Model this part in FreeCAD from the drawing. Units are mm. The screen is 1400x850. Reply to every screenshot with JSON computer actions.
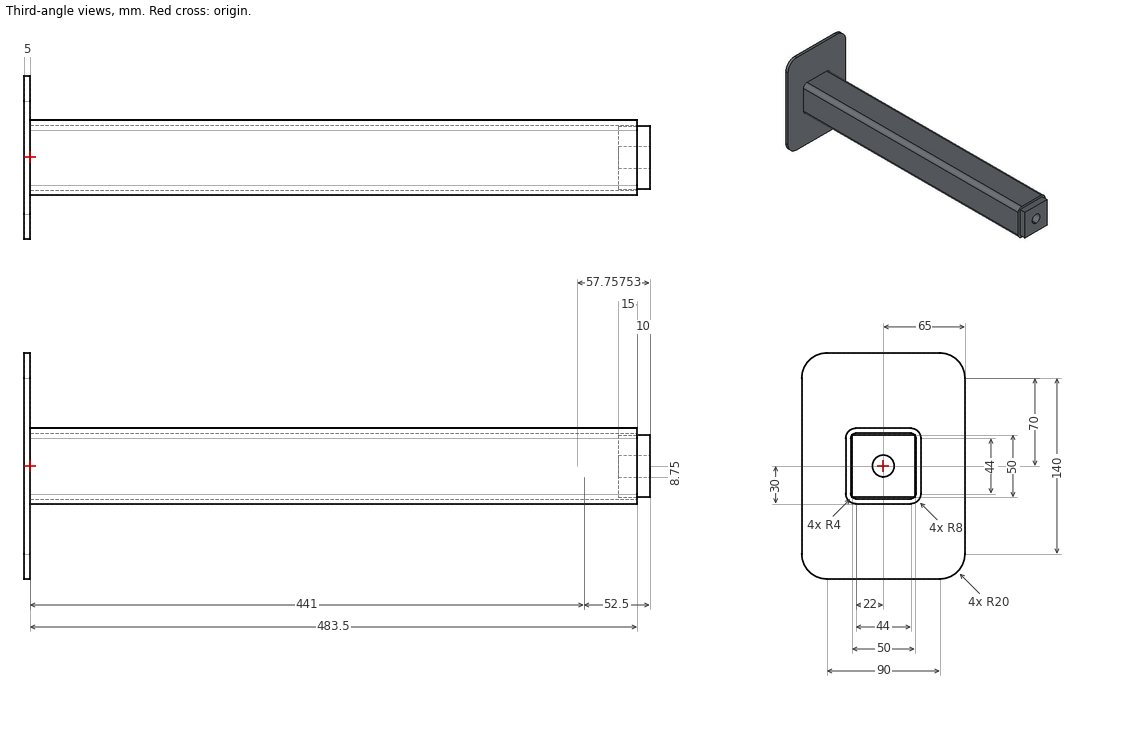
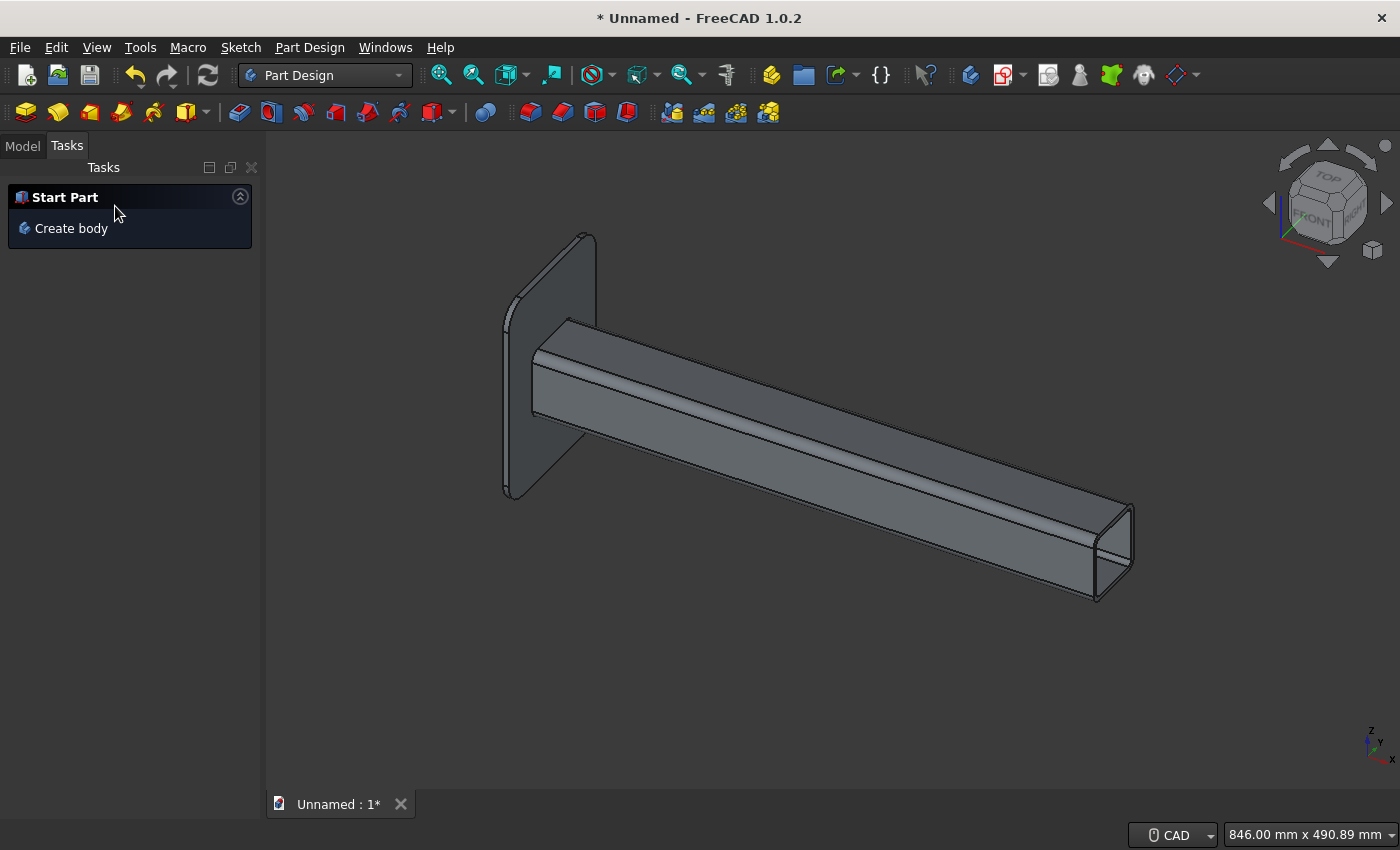
{"action": "left_click", "coordinate": [442, 76]}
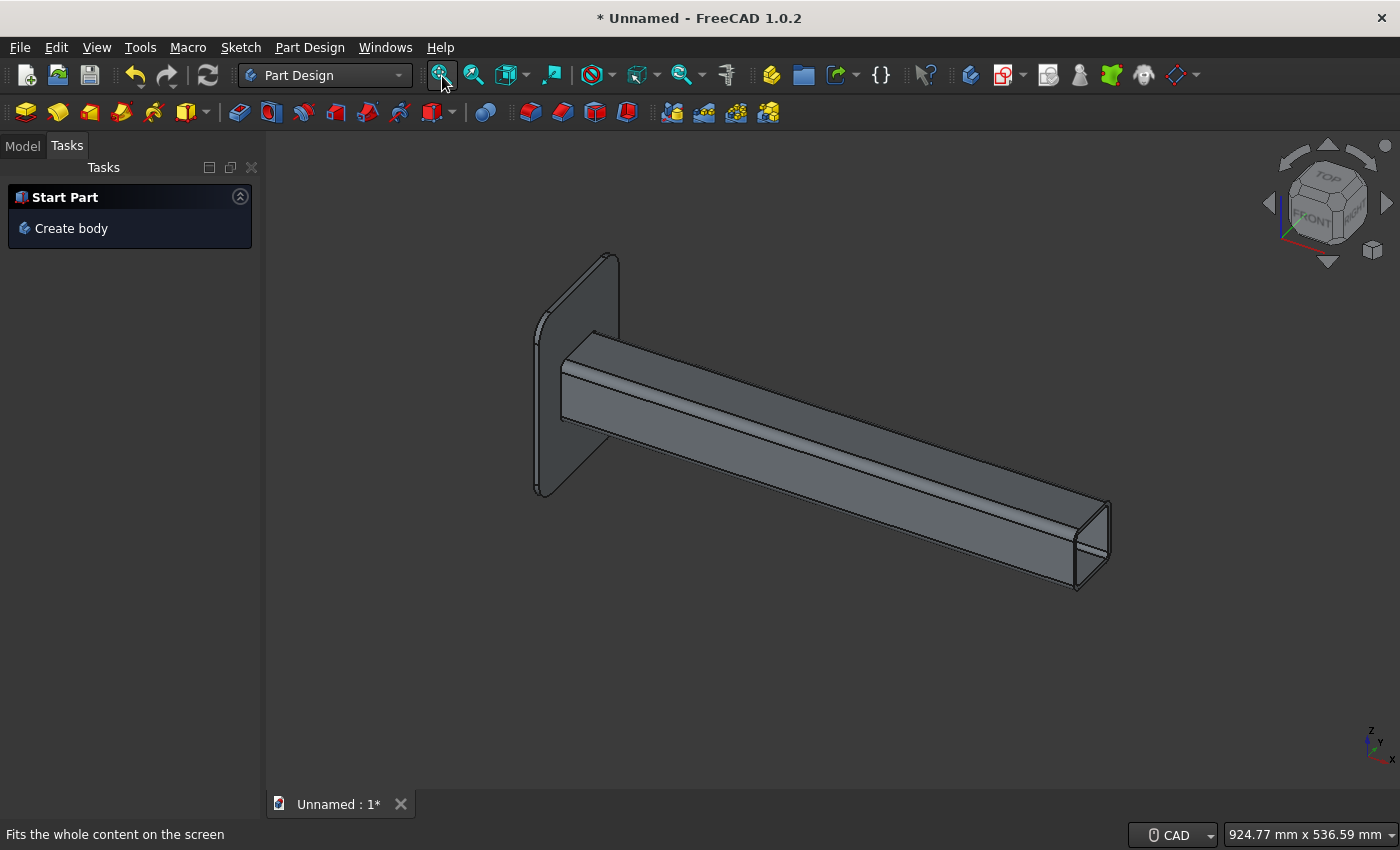
{"action": "left_click", "coordinate": [972, 76]}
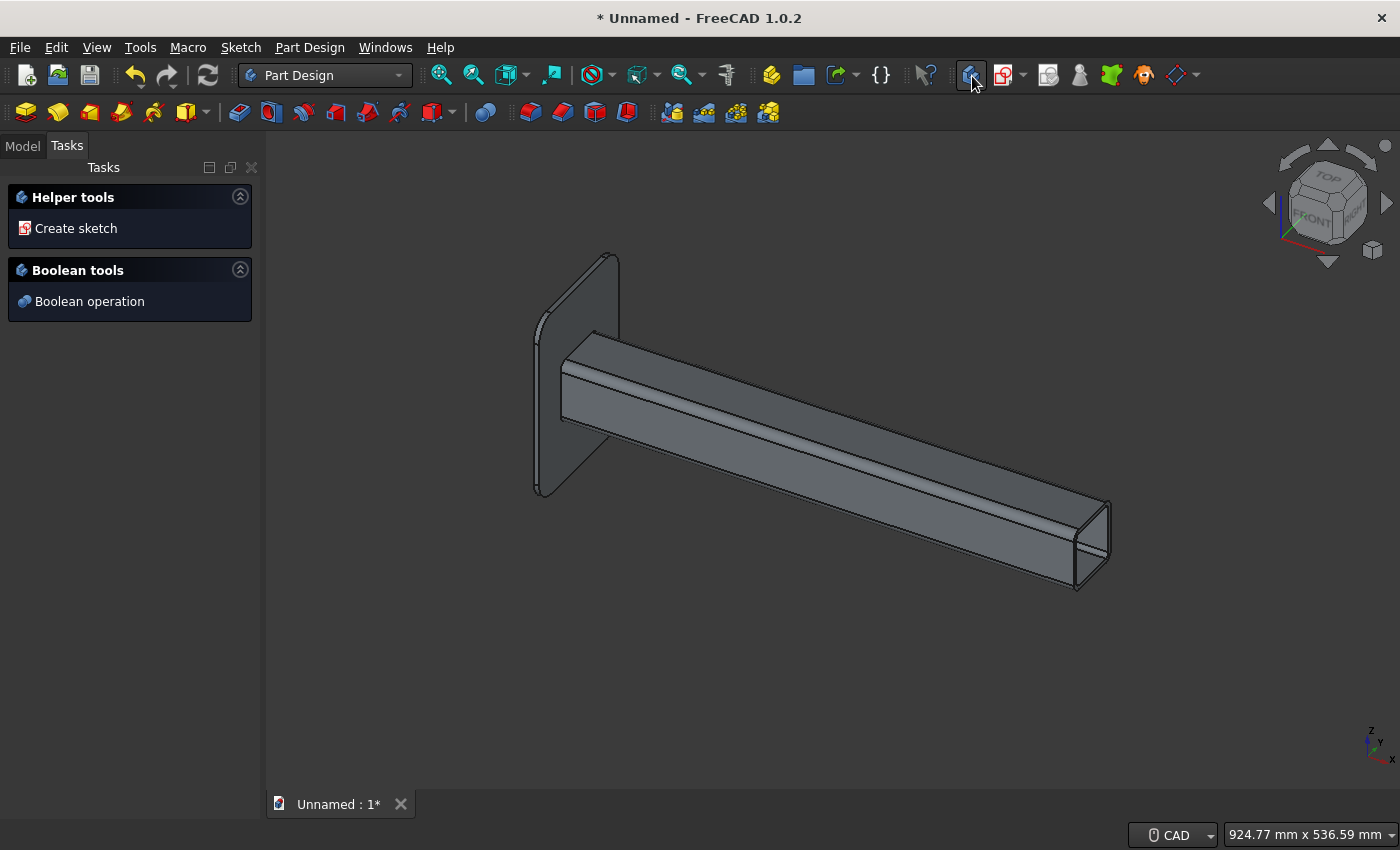
{"action": "left_click", "coordinate": [23, 145]}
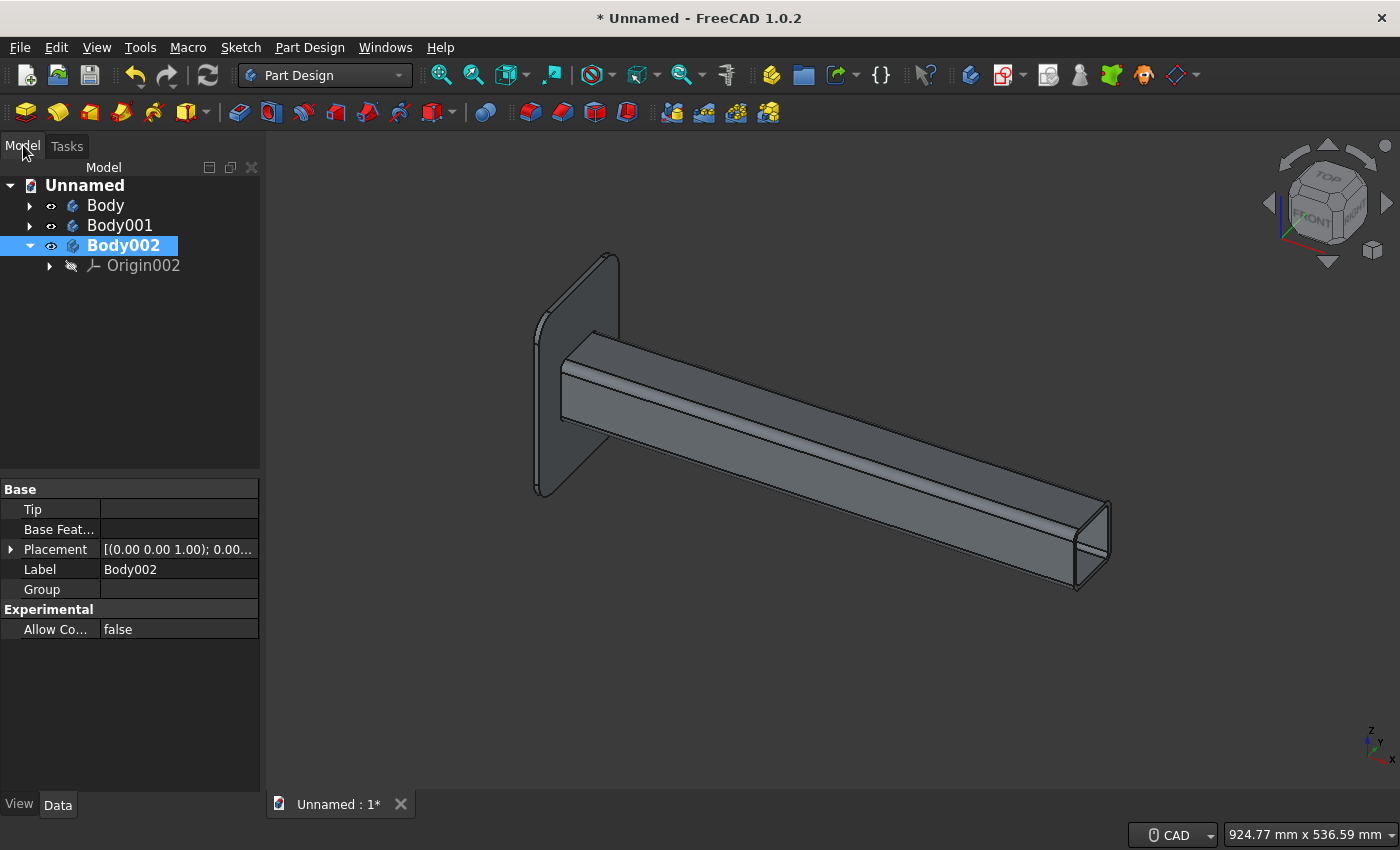
{"action": "left_click", "coordinate": [50, 266]}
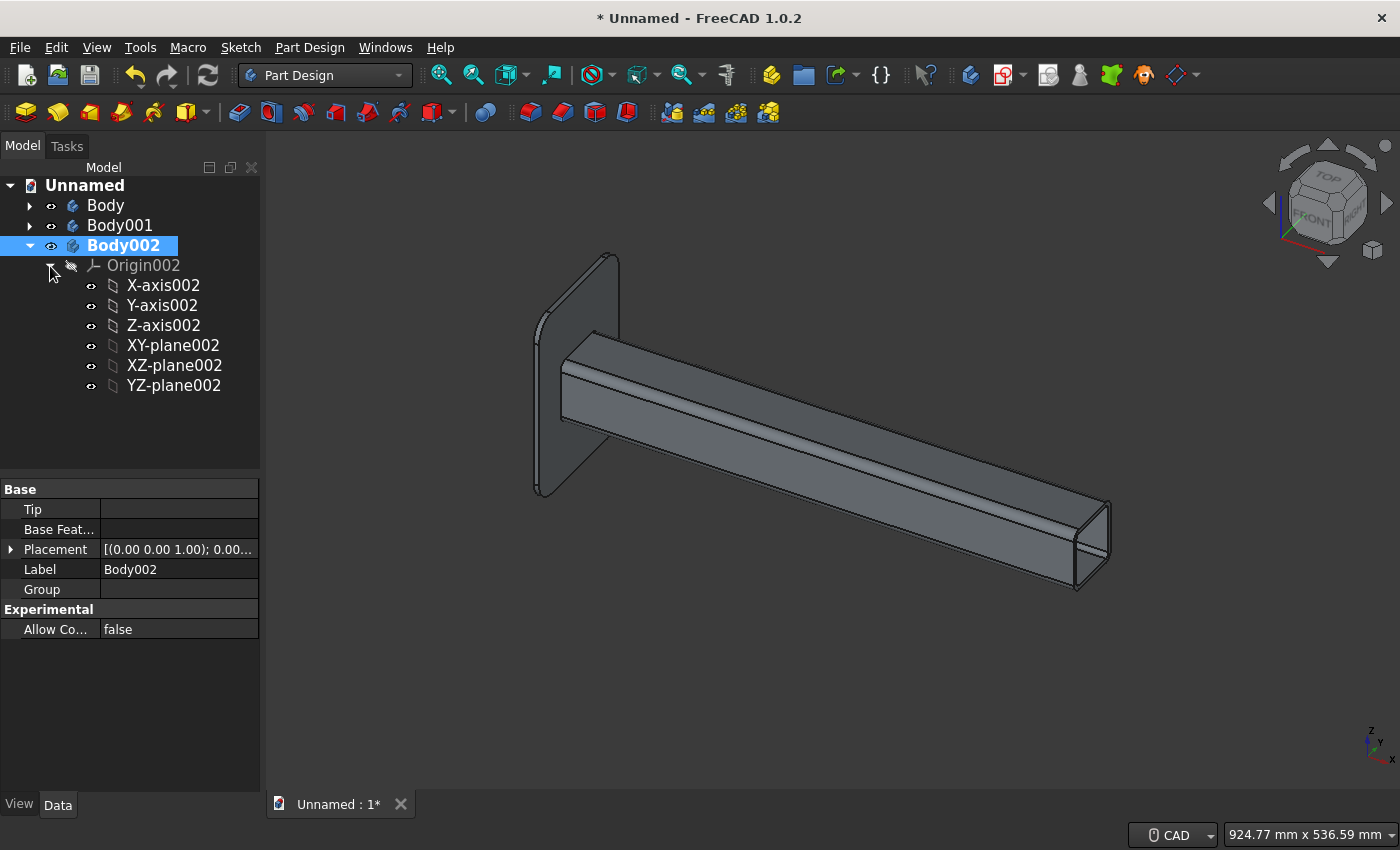
{"action": "left_click", "coordinate": [136, 386]}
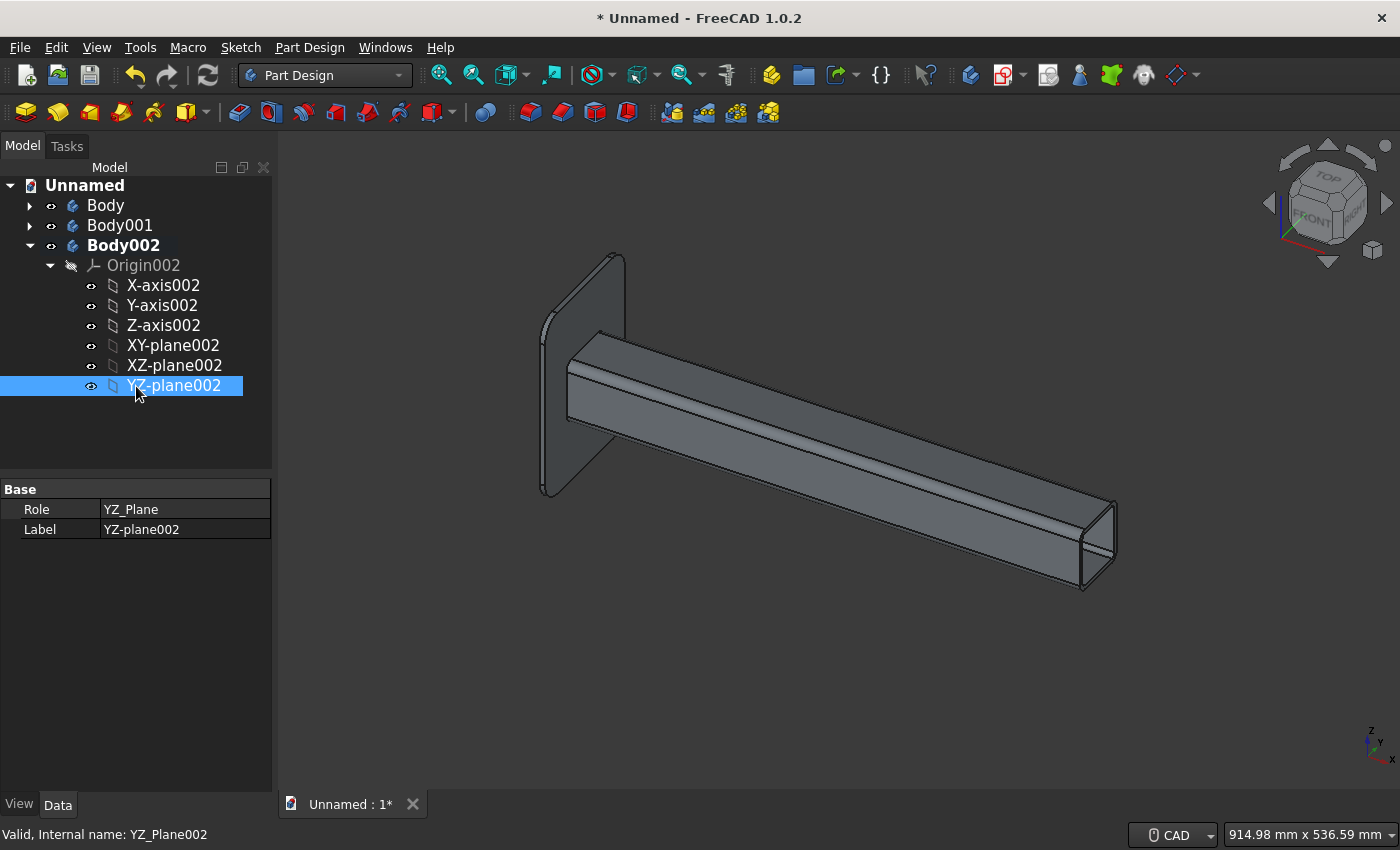
{"action": "left_click", "coordinate": [1176, 76]}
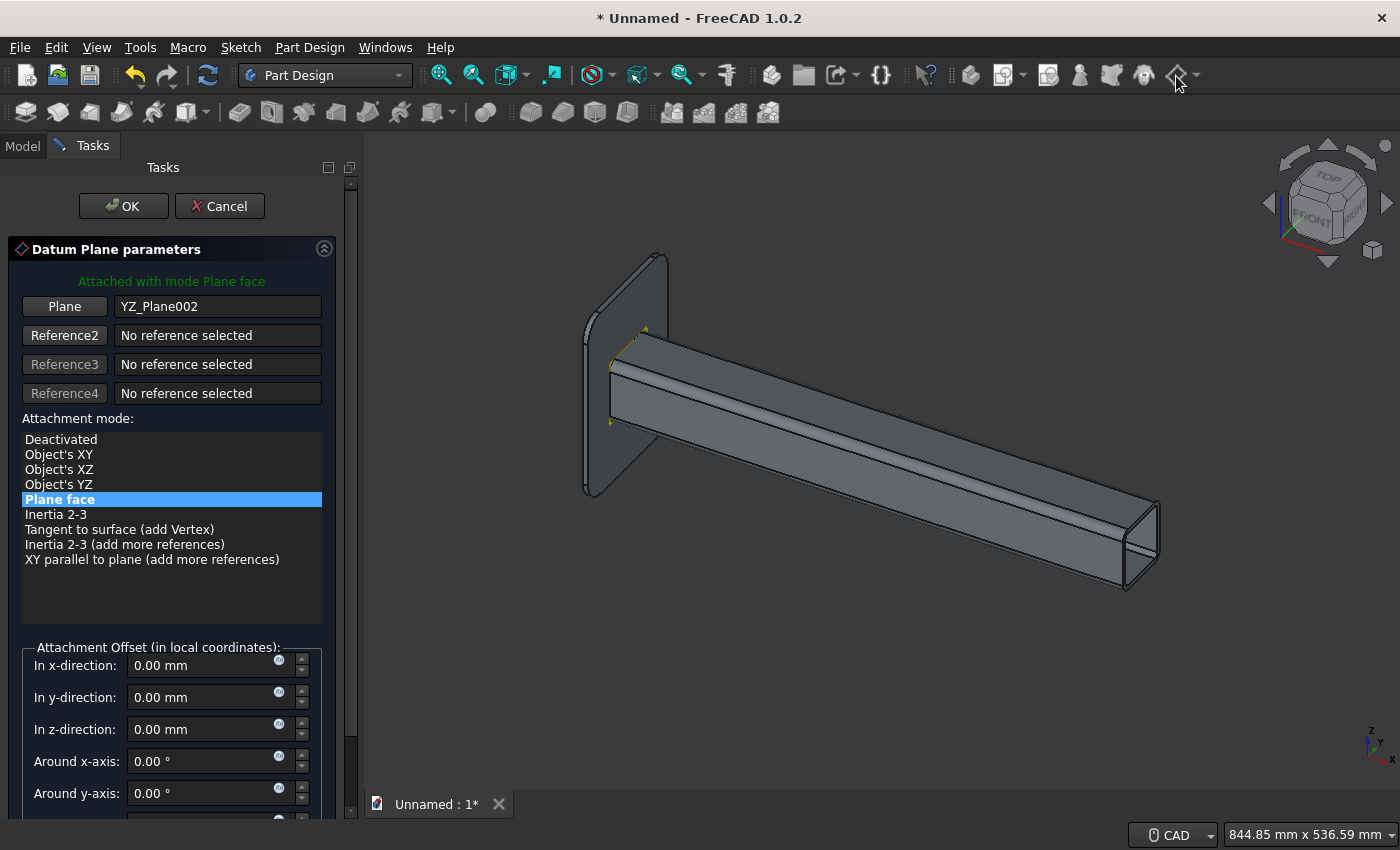
{"action": "triple_click", "coordinate": [210, 729]}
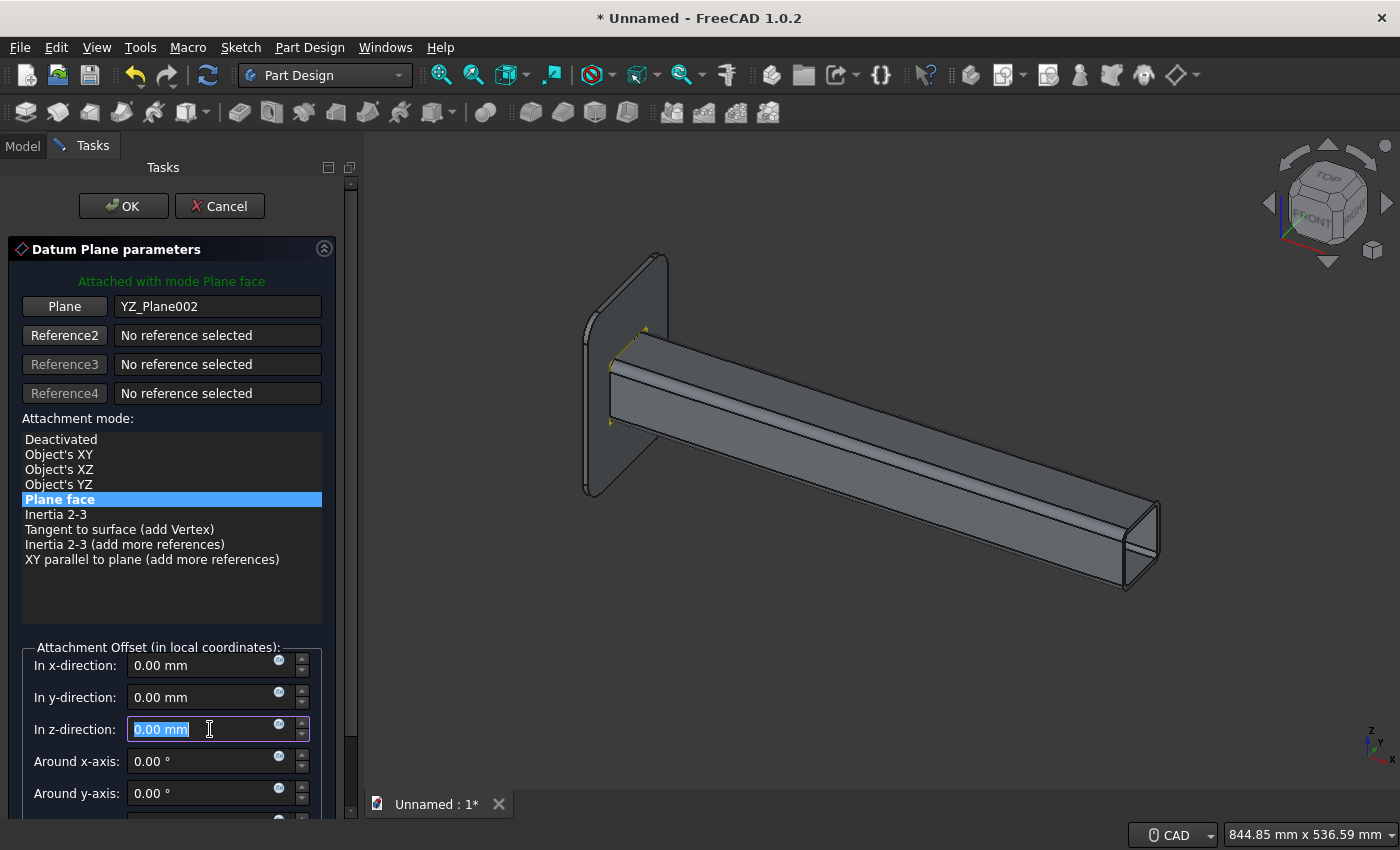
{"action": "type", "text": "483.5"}
{"action": "key", "text": "Tab"}